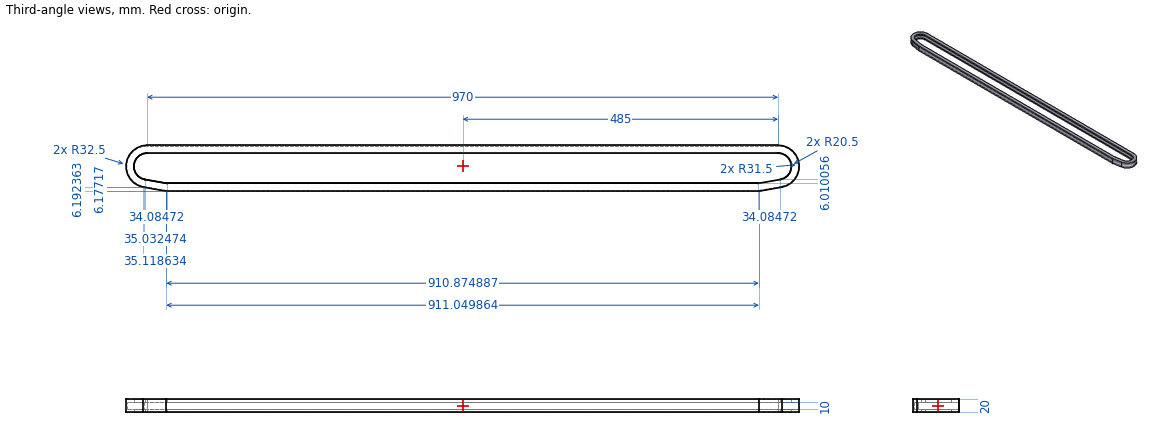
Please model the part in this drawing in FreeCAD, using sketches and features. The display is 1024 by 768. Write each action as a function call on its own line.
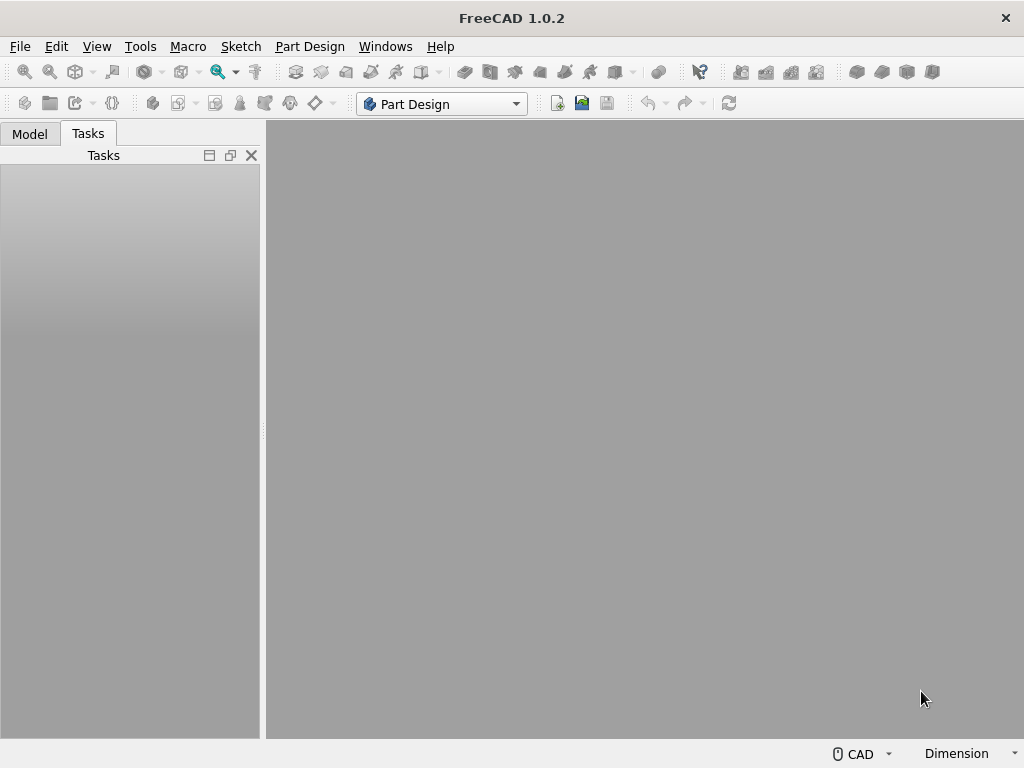
key(ctrl+n)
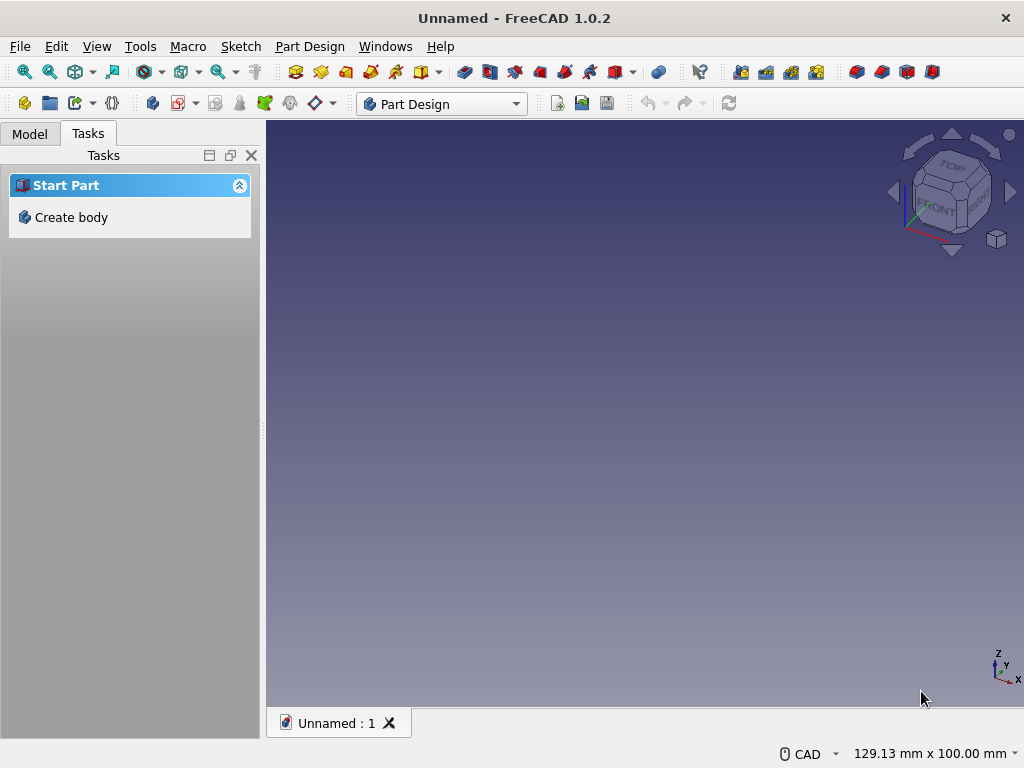
click(178, 104)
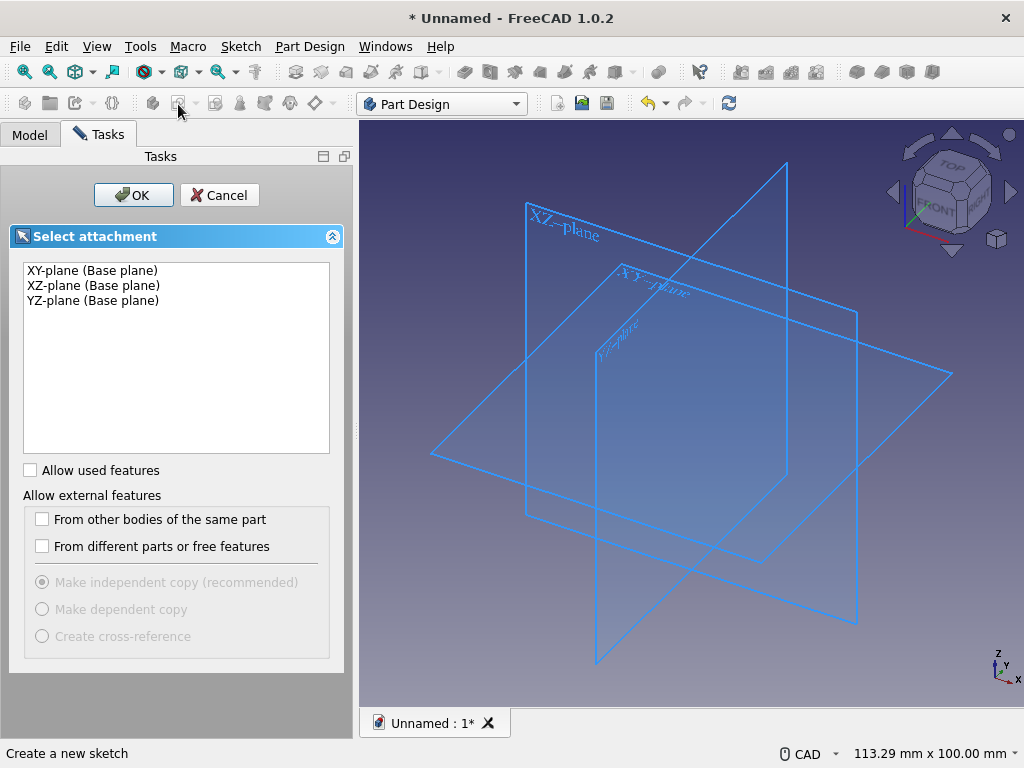
click(84, 270)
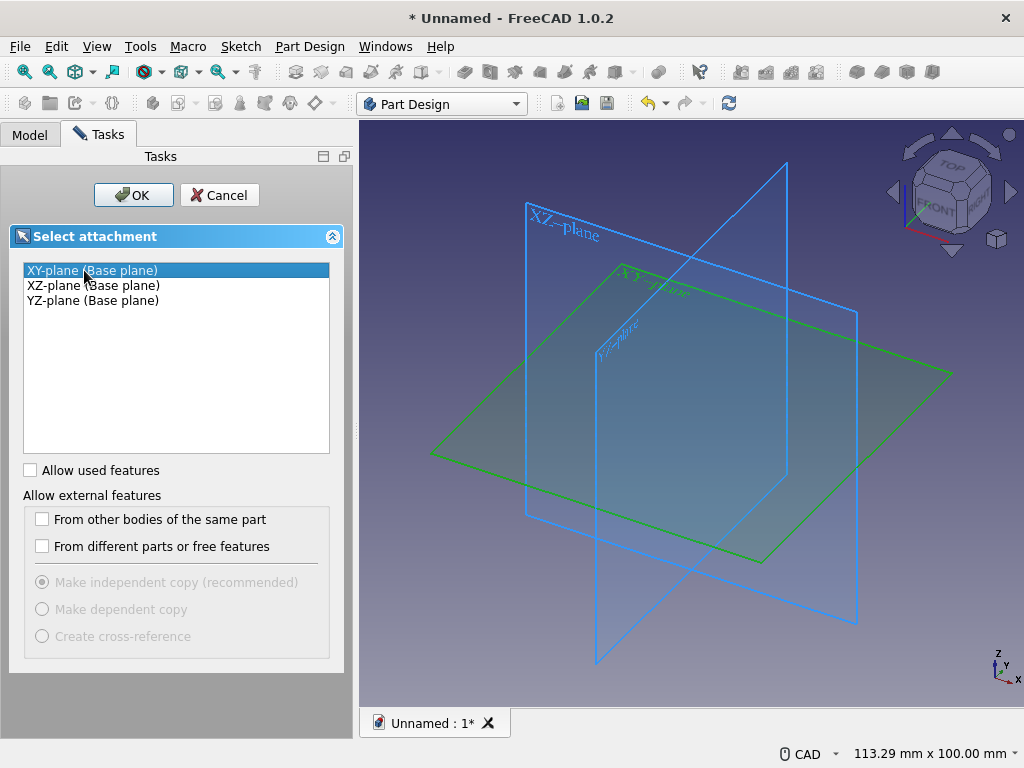
click(134, 195)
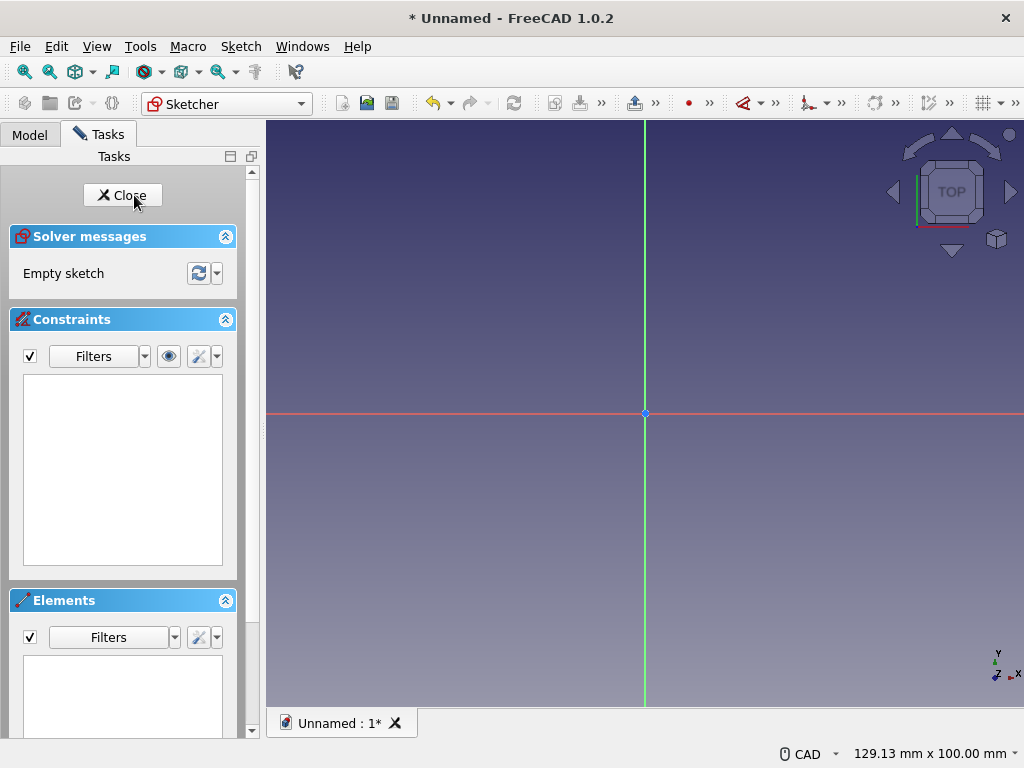
scroll(572, 412, down, 14)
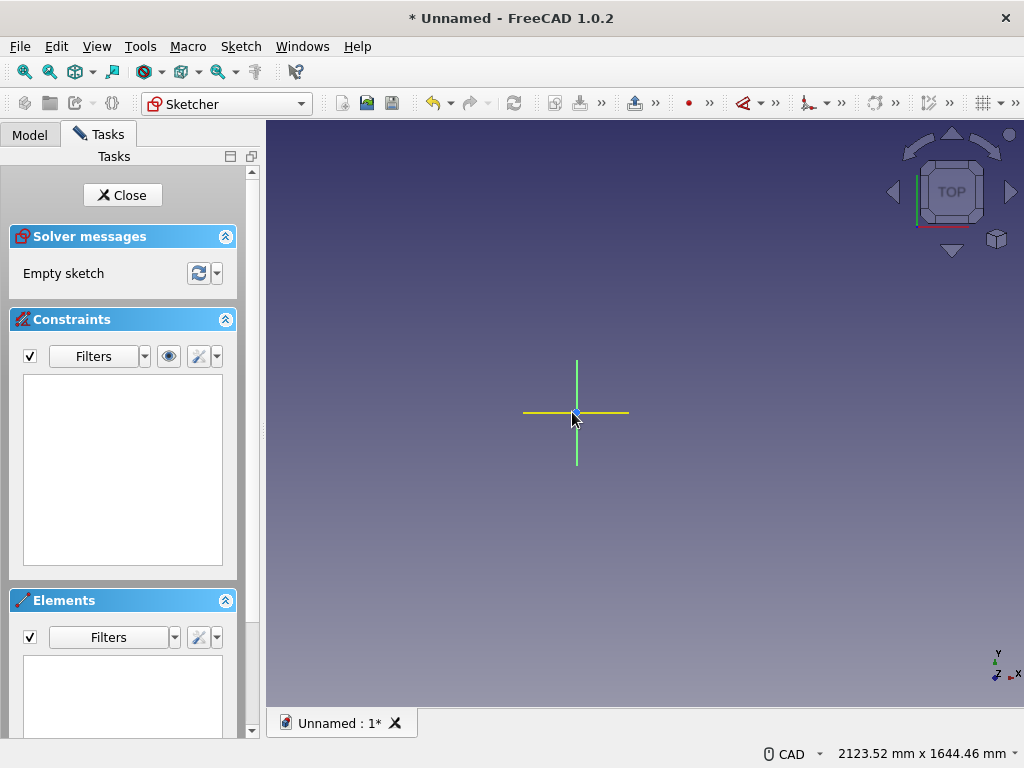
key(g)
key(l)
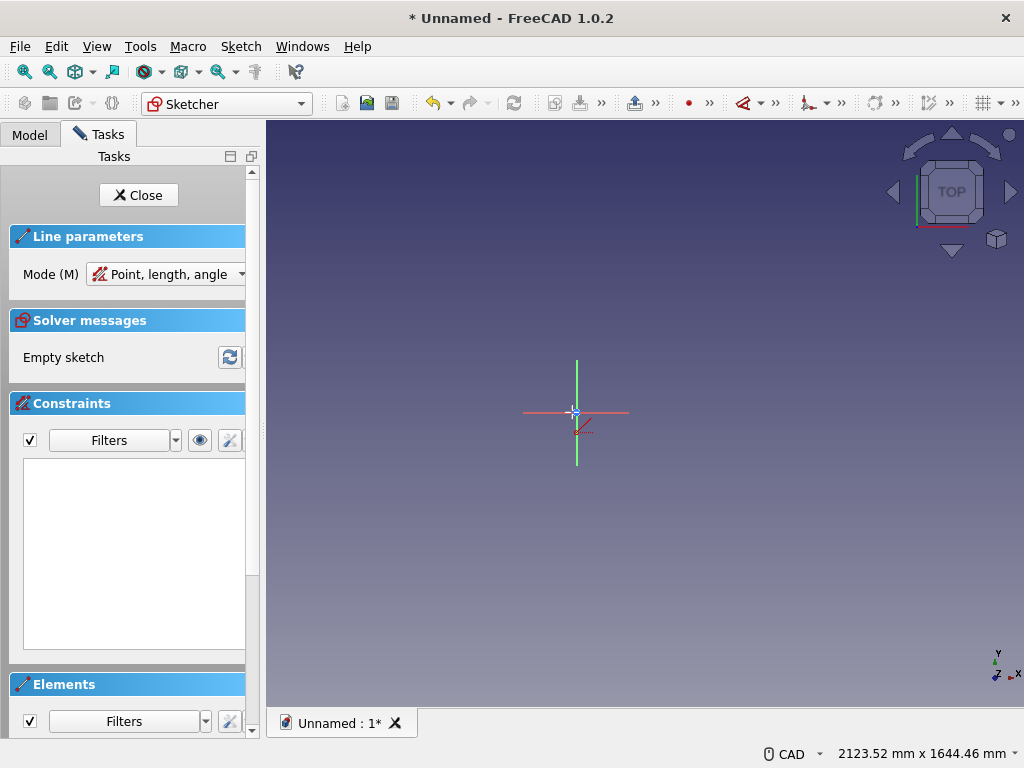
scroll(750, 401, up, 2)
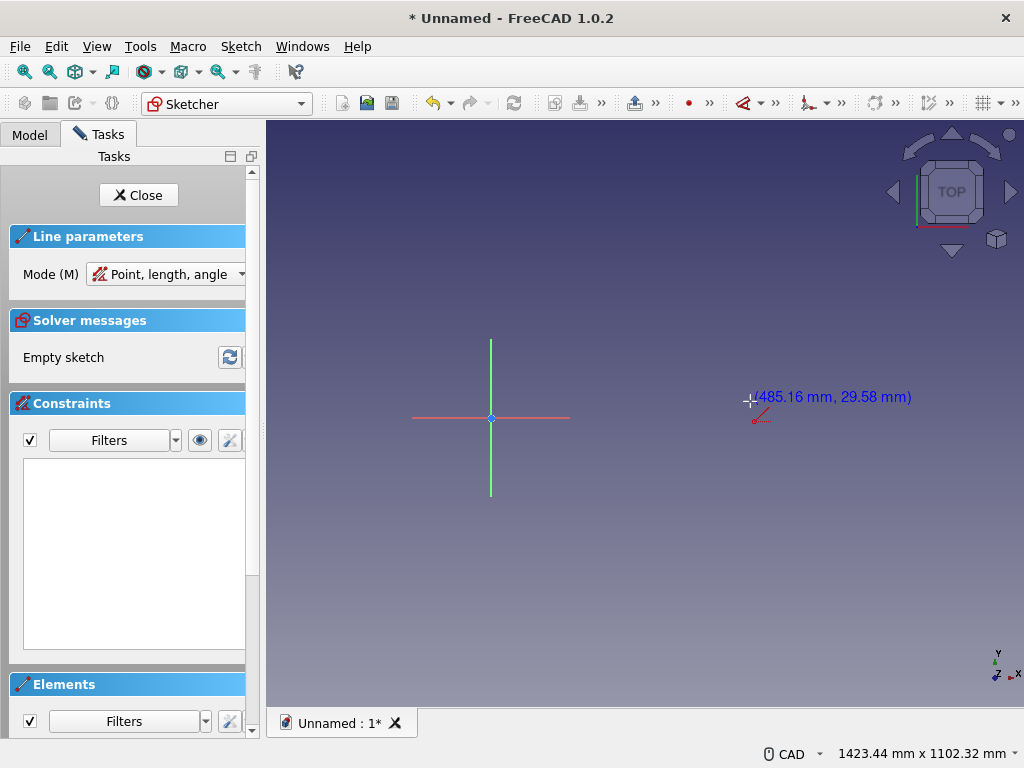
click(750, 401)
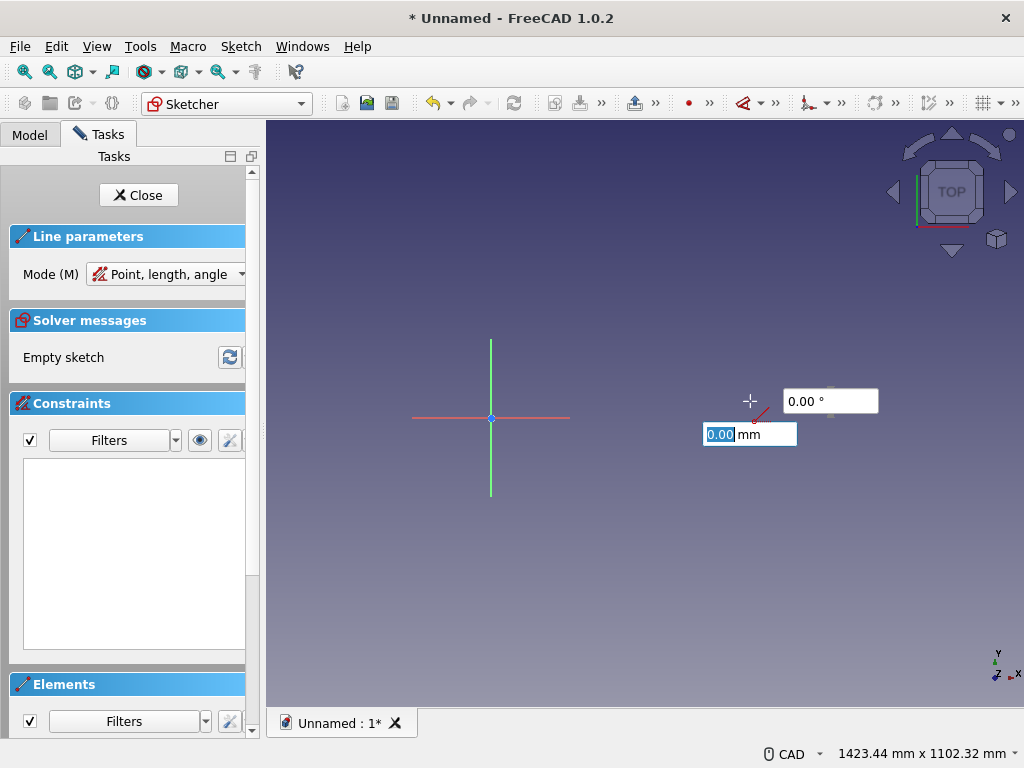
scroll(750, 401, down, 2)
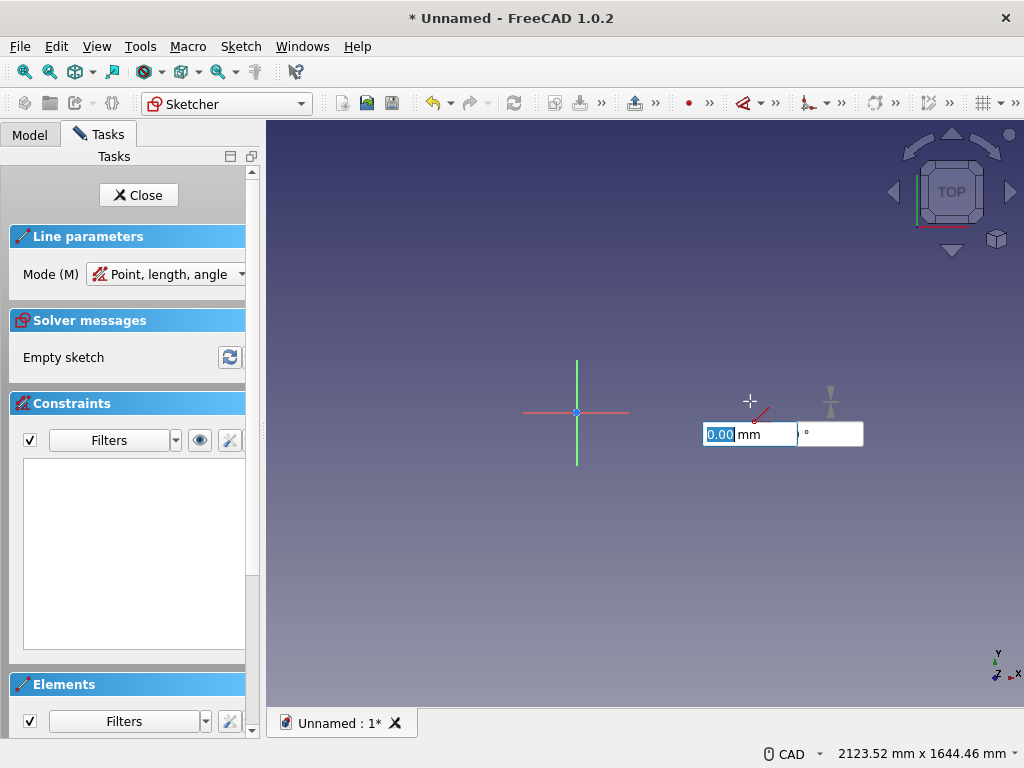
scroll(404, 401, up, 2)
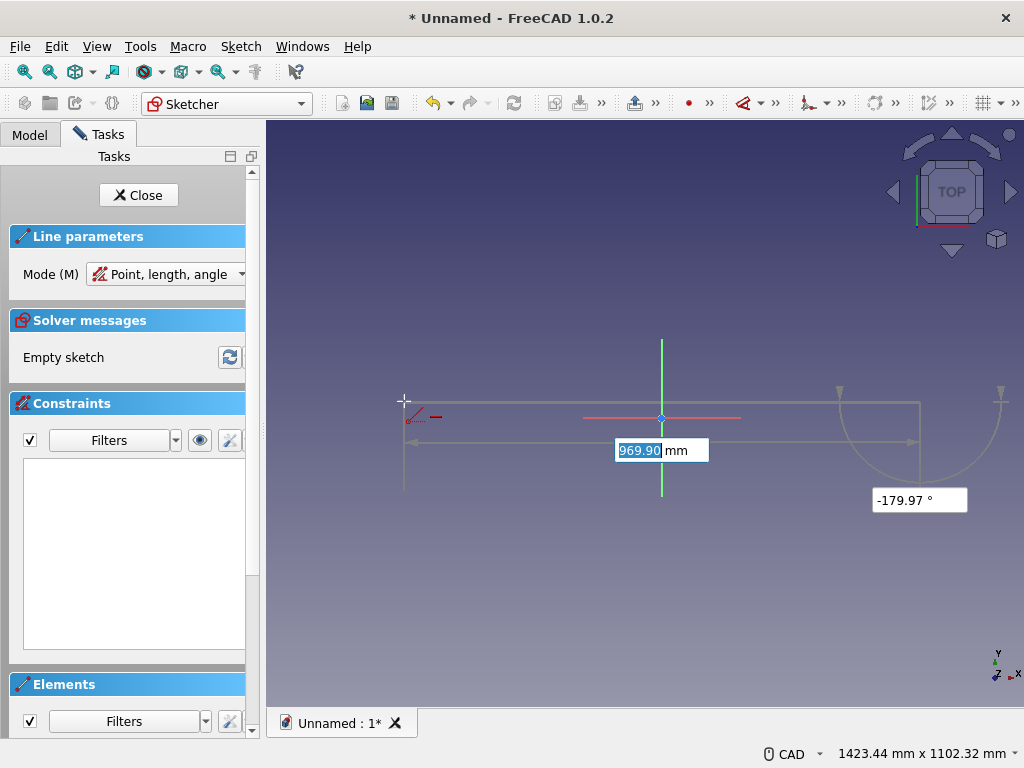
click(403, 401)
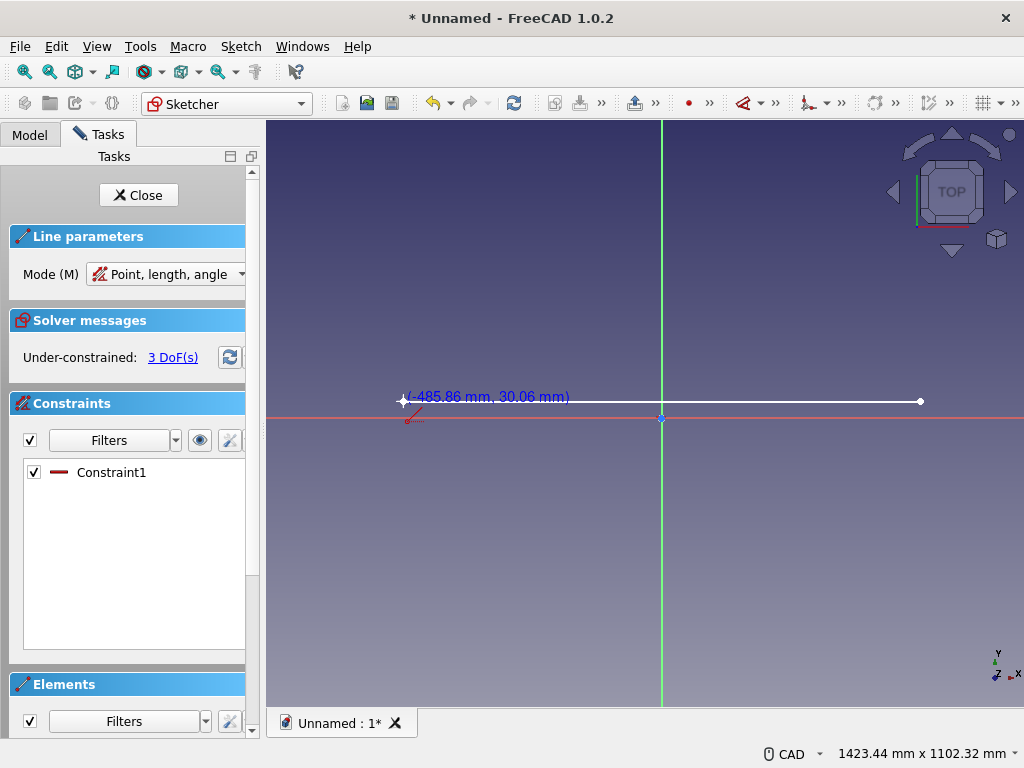
key(g)
key(m)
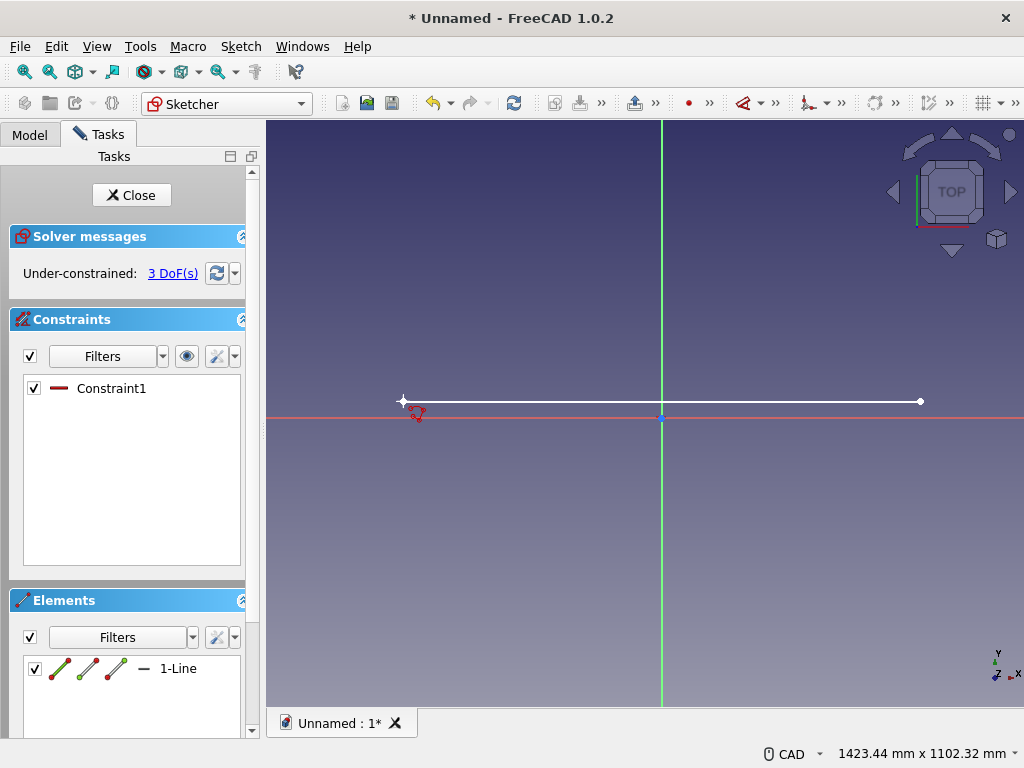
click(400, 435)
click(419, 438)